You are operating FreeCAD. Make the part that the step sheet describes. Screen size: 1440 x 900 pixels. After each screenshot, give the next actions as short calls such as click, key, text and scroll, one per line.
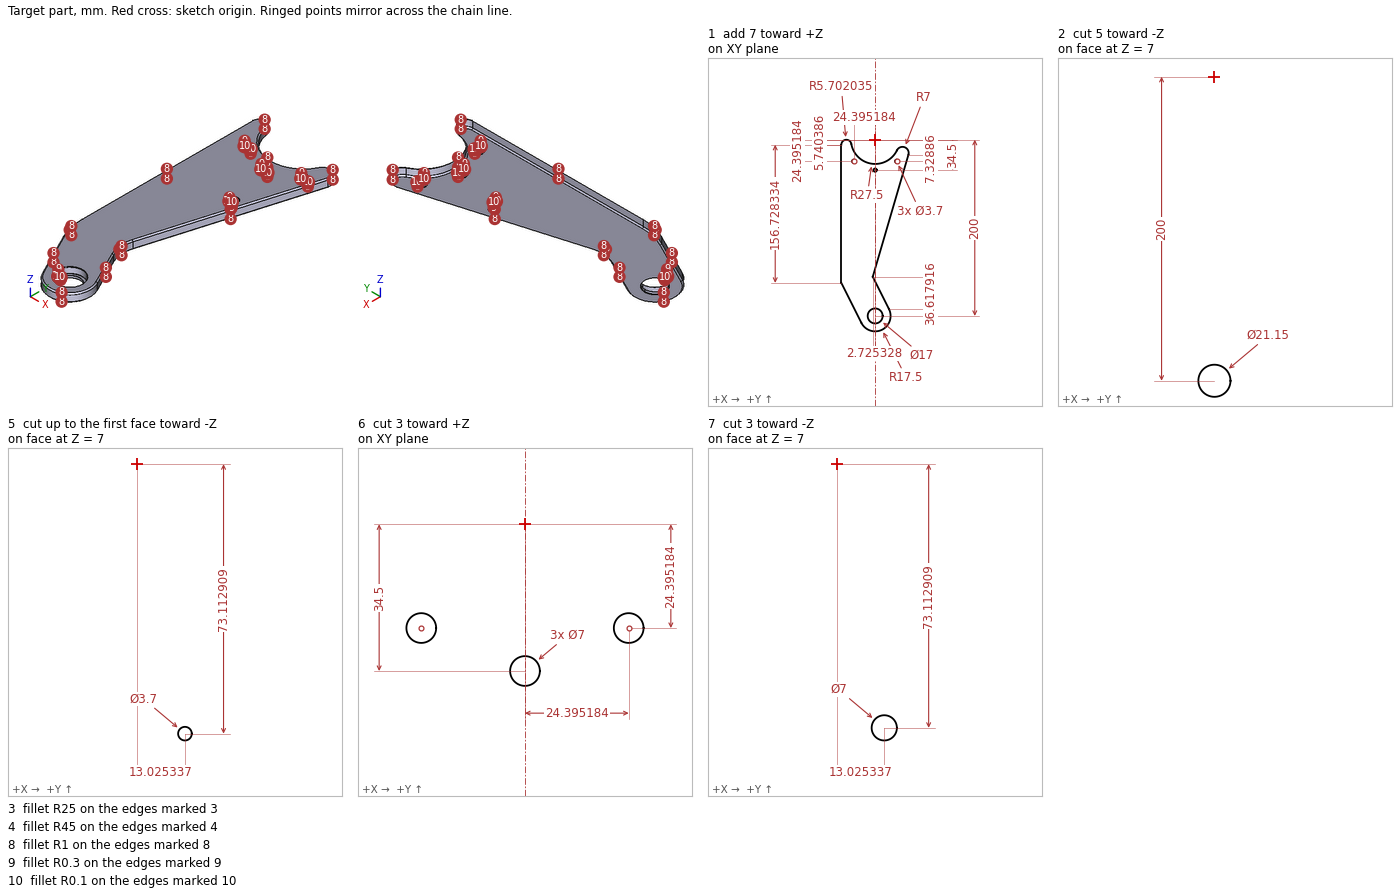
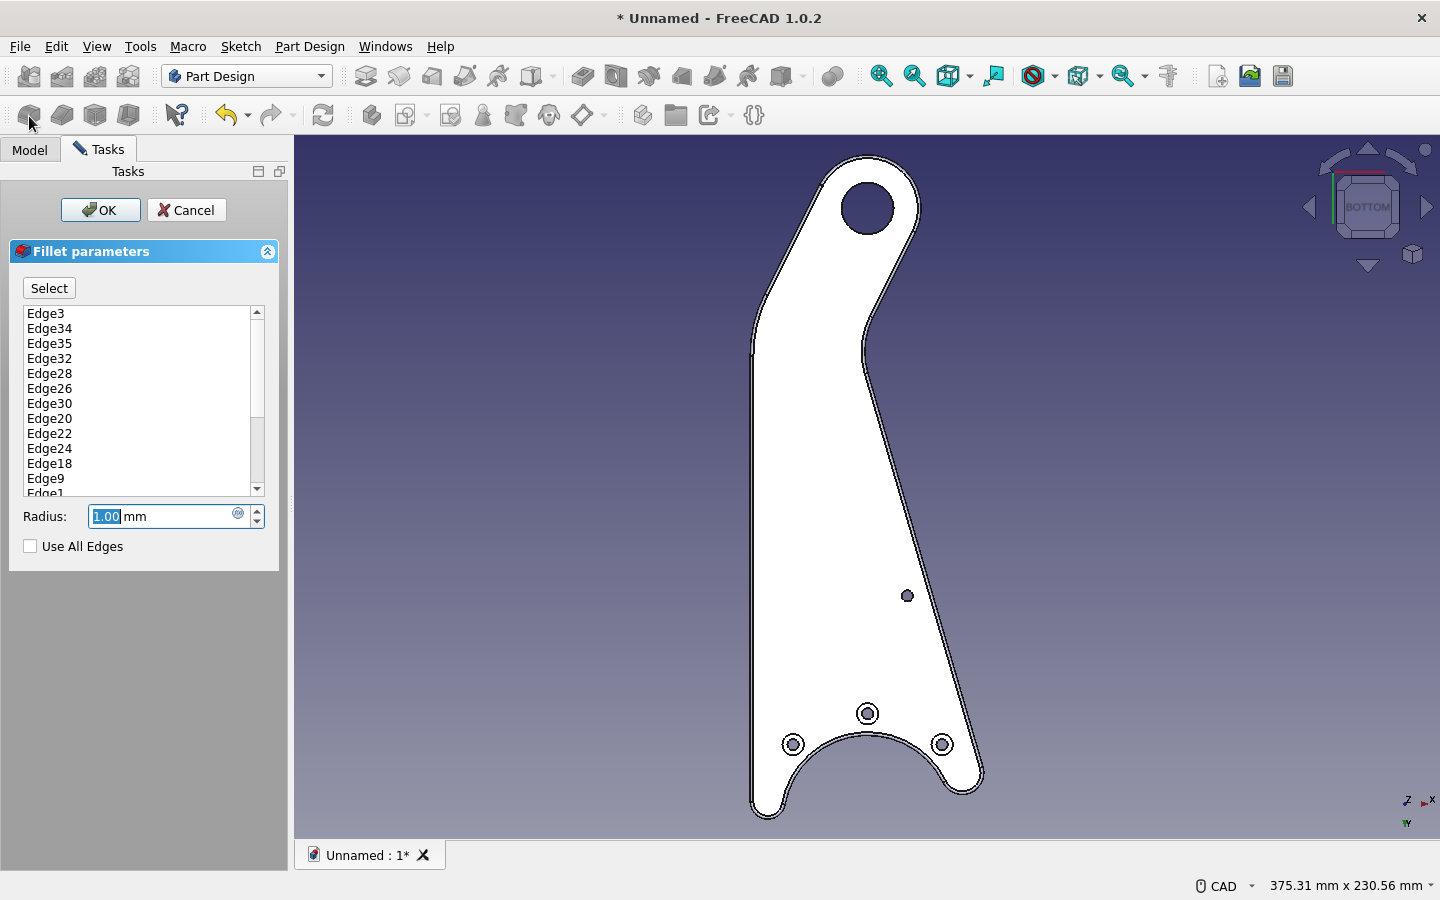
text(1)
key(Tab)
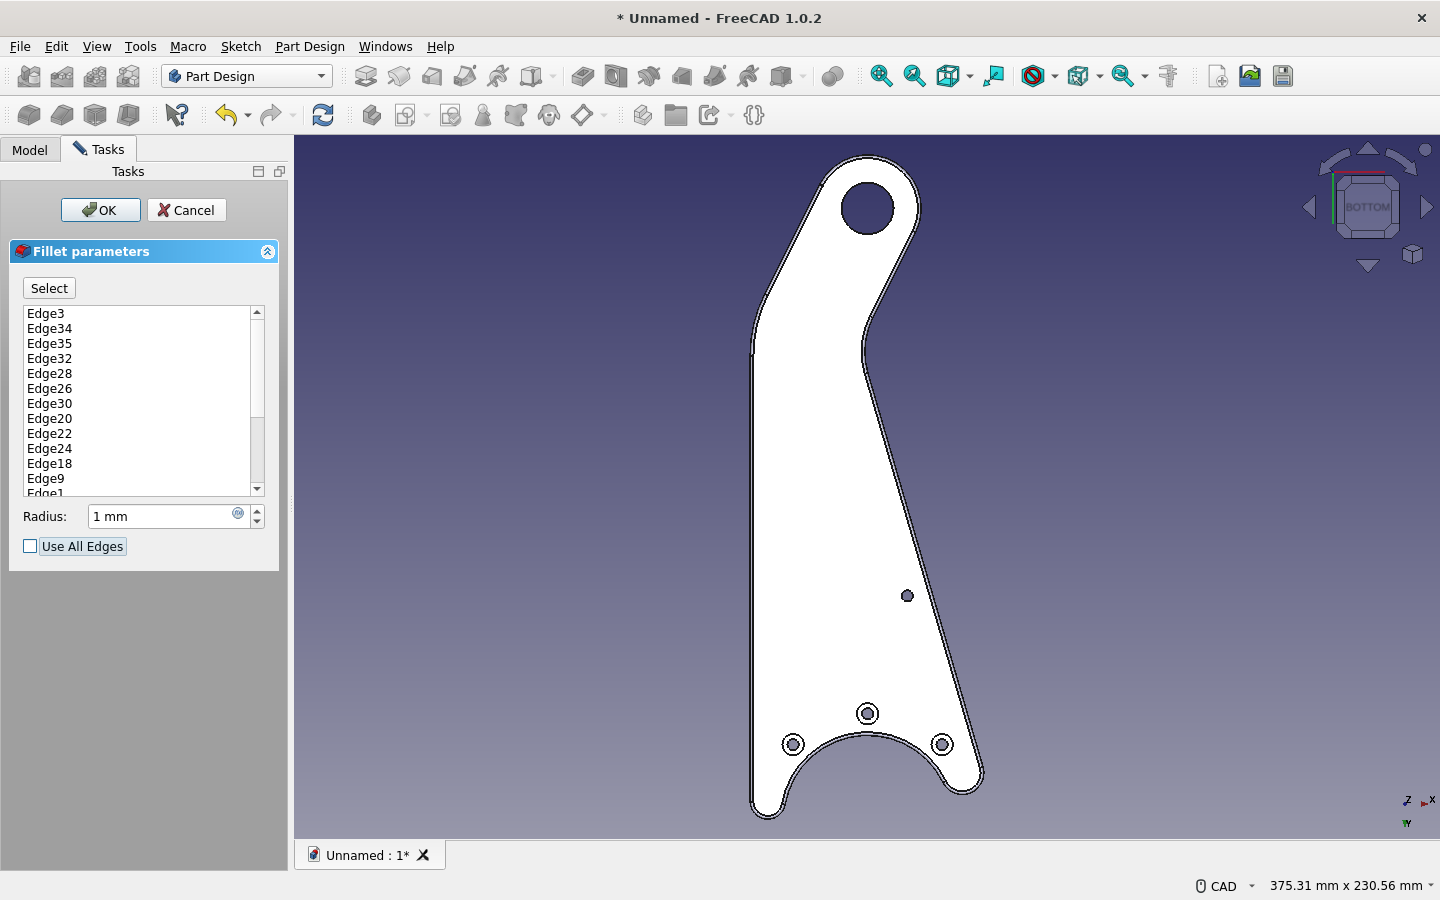
click(101, 210)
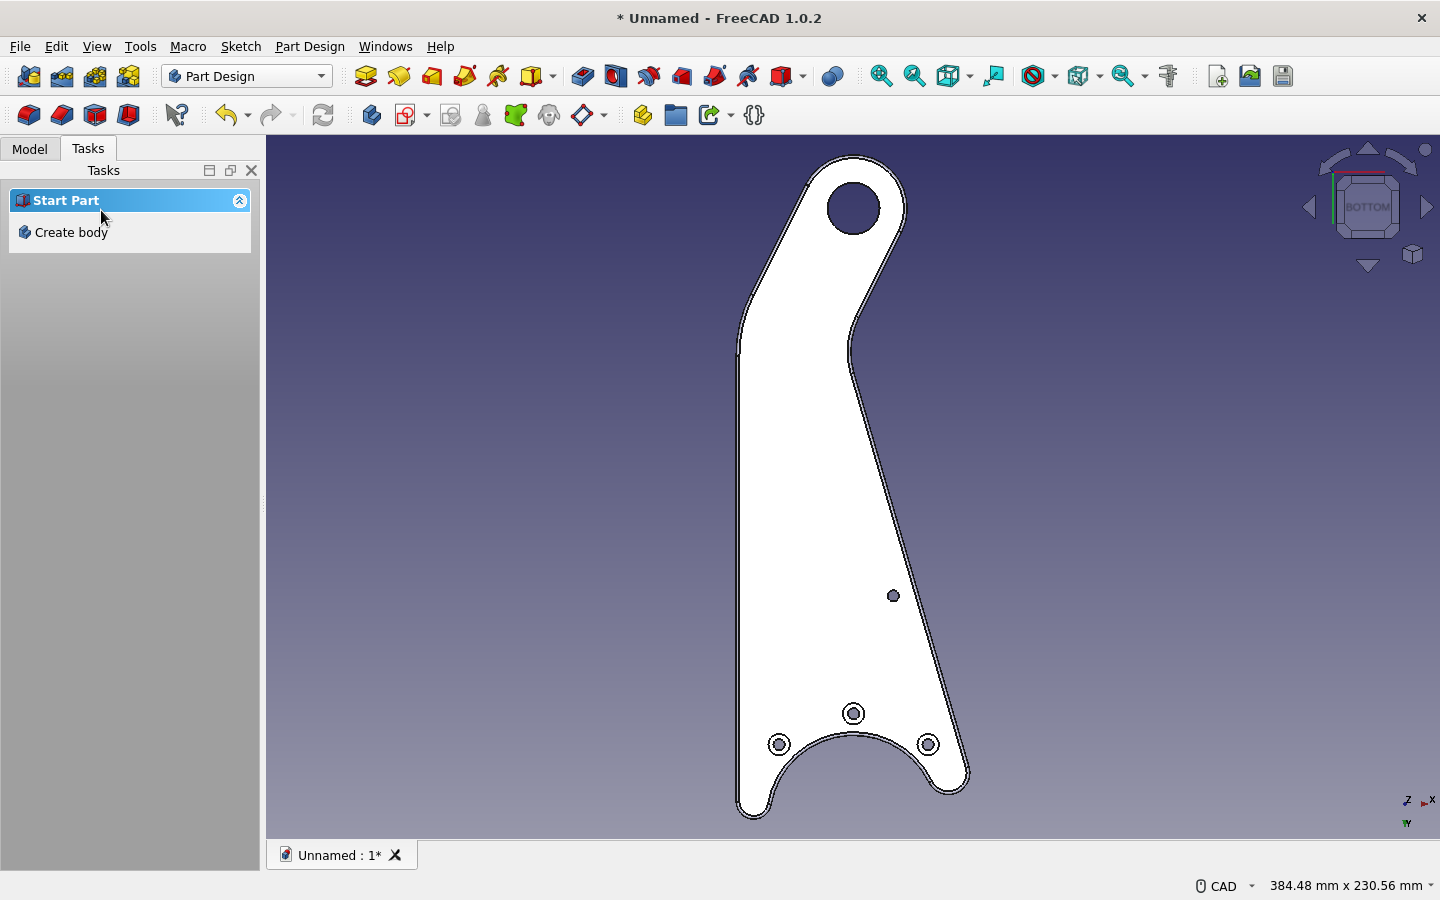
click(846, 232)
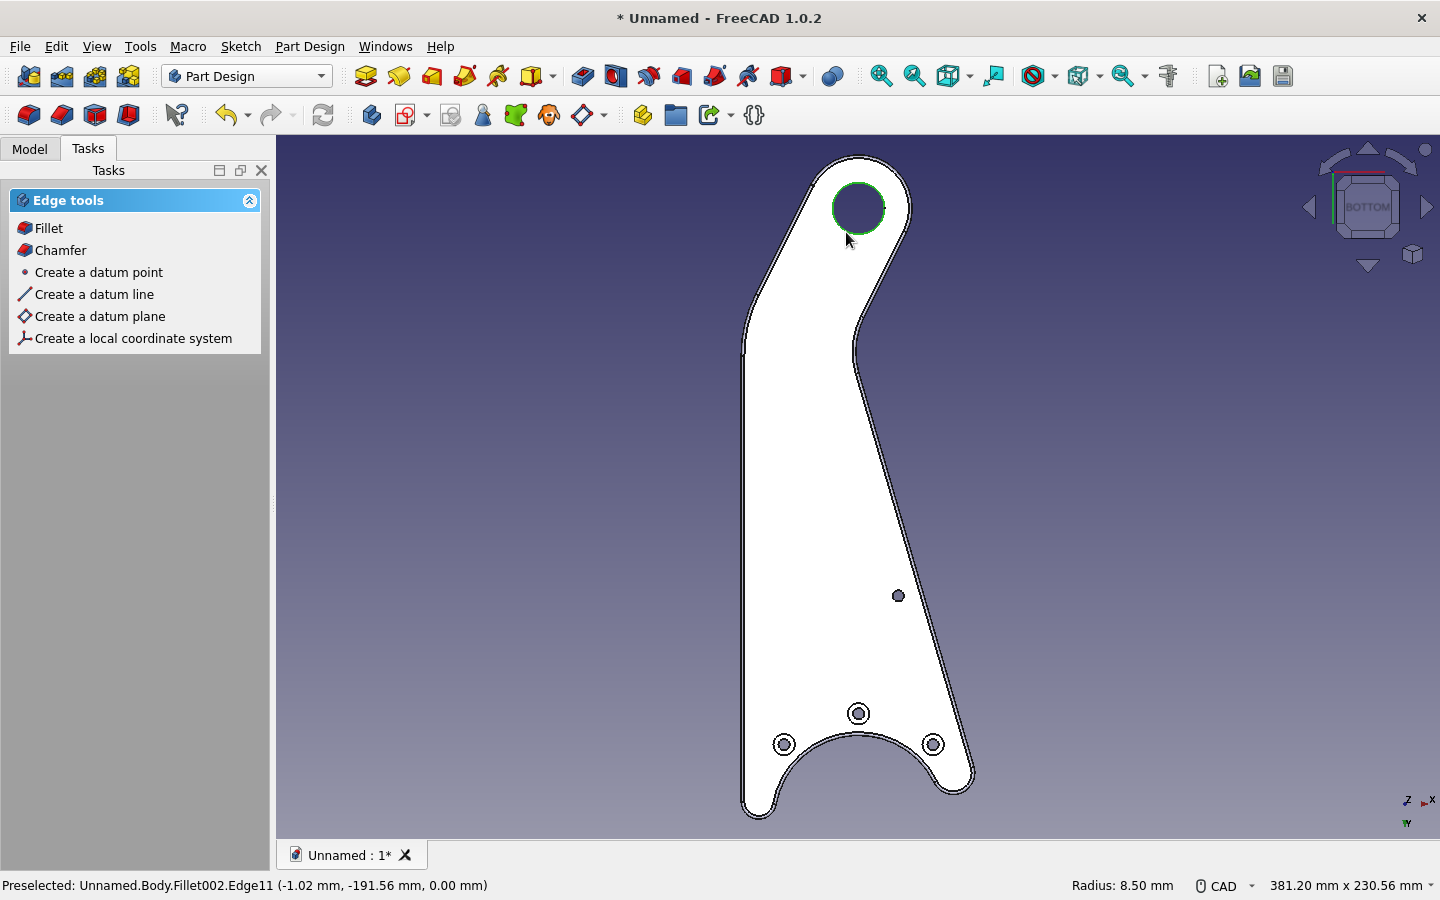
click(893, 595, ctrl)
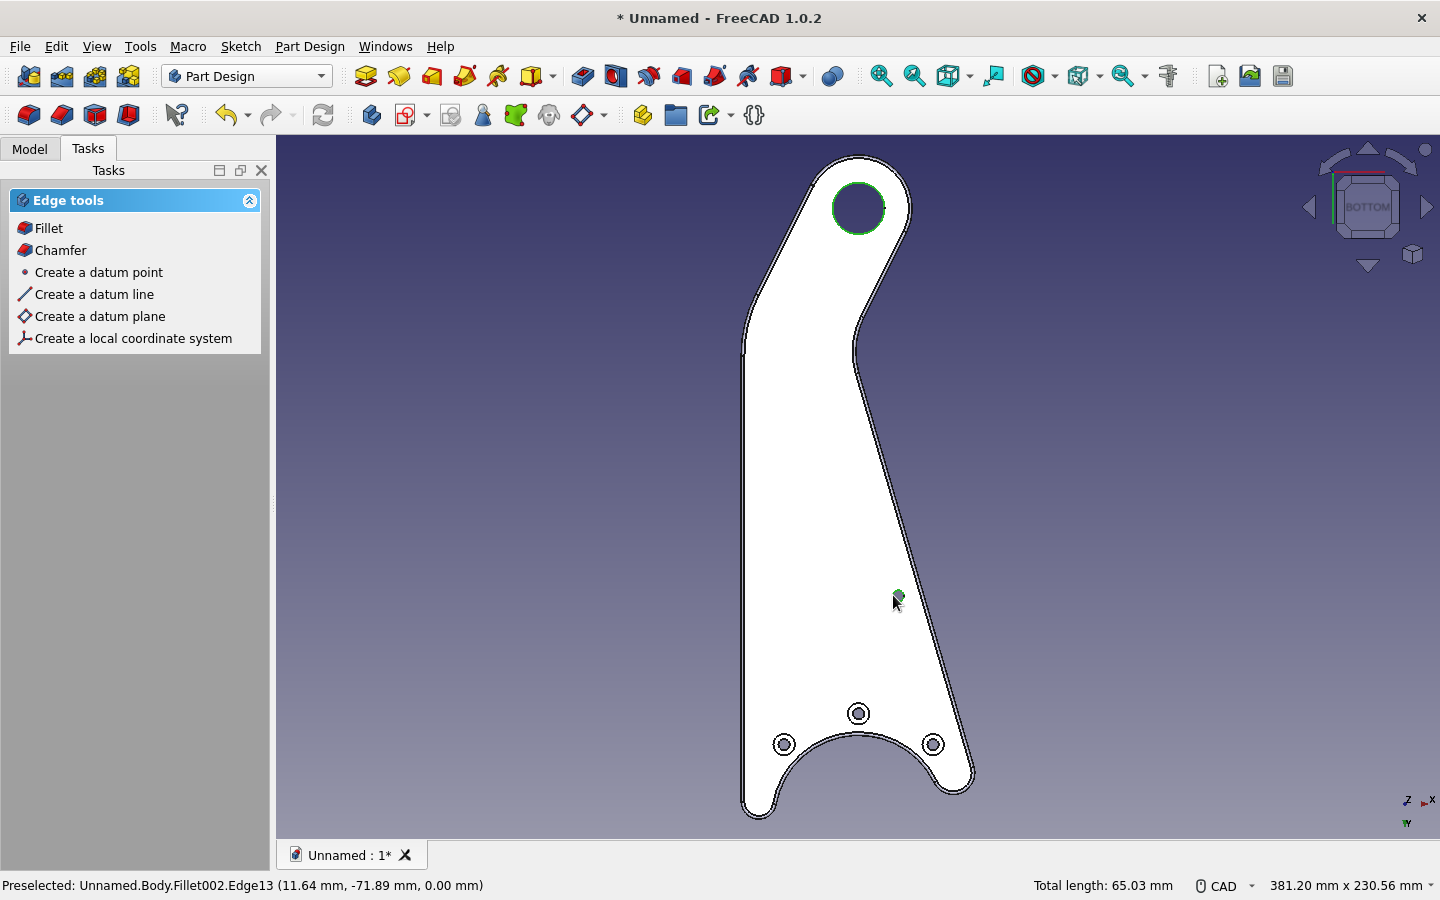
click(850, 719, ctrl)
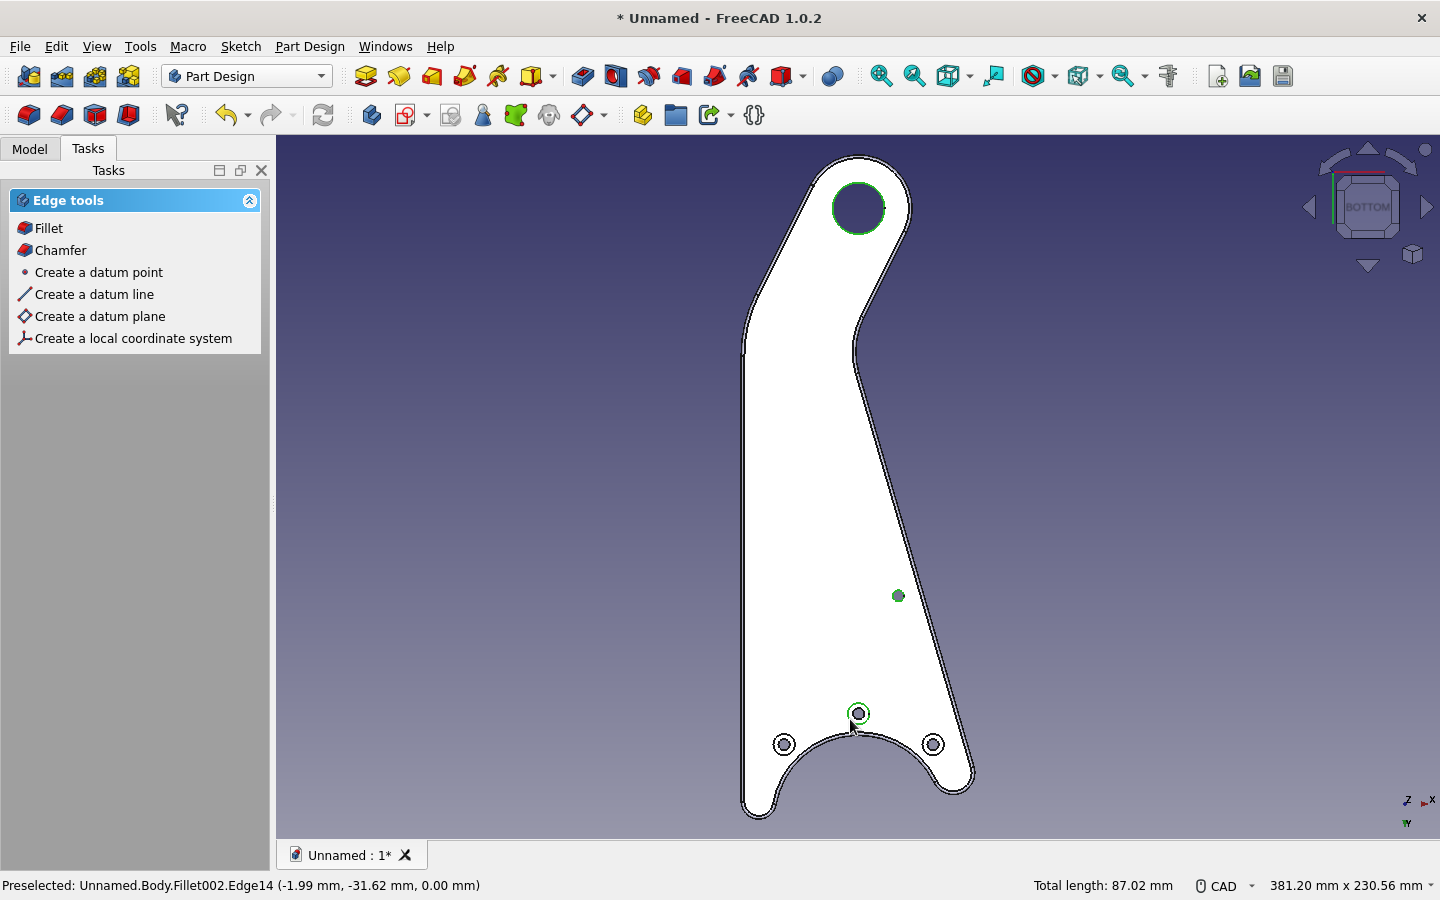
click(924, 750, ctrl)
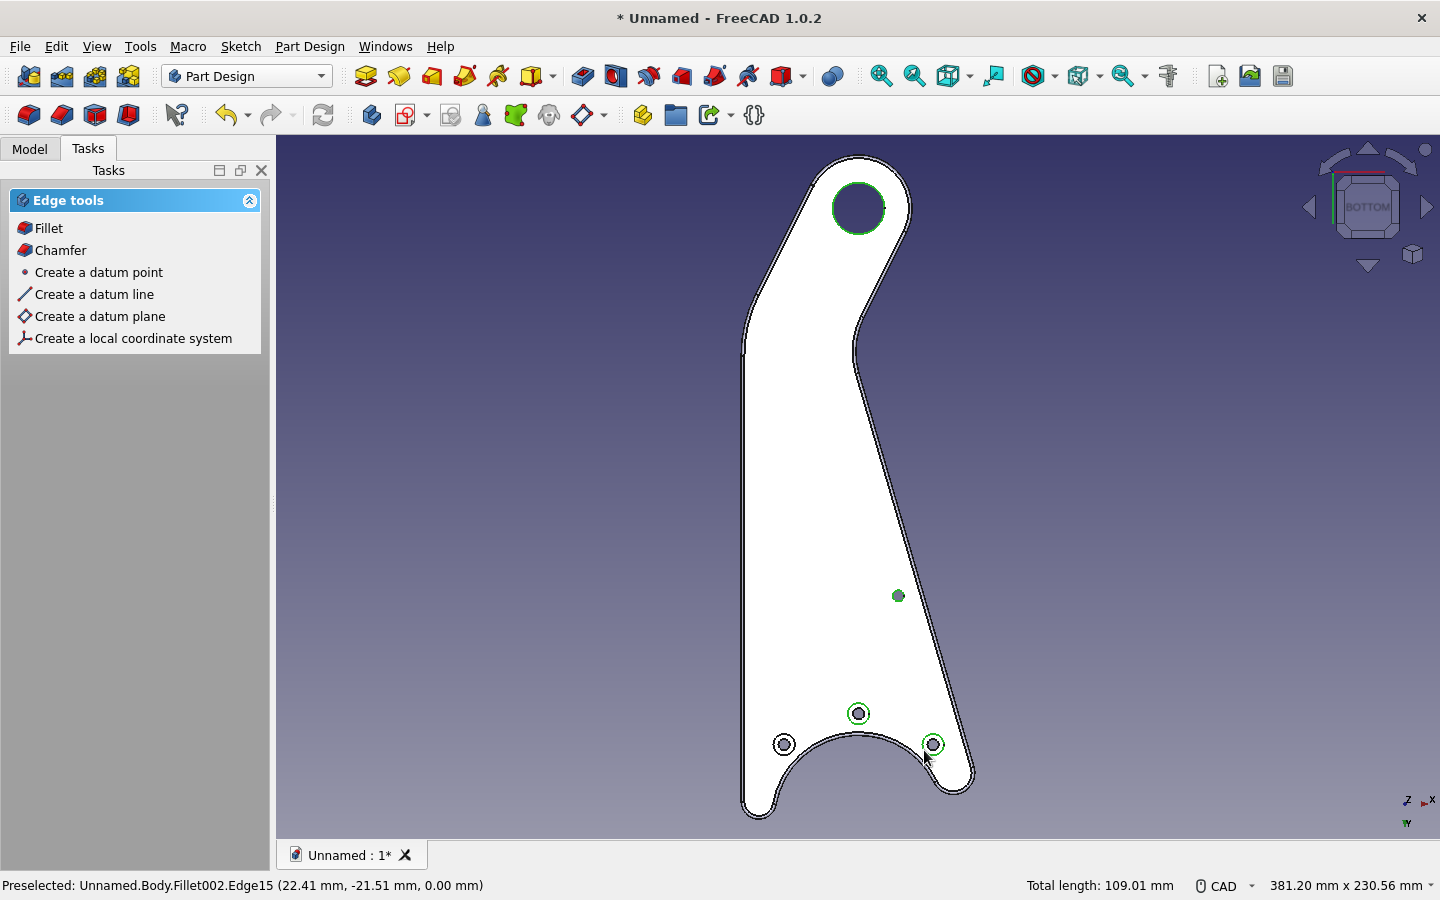
click(775, 750, ctrl)